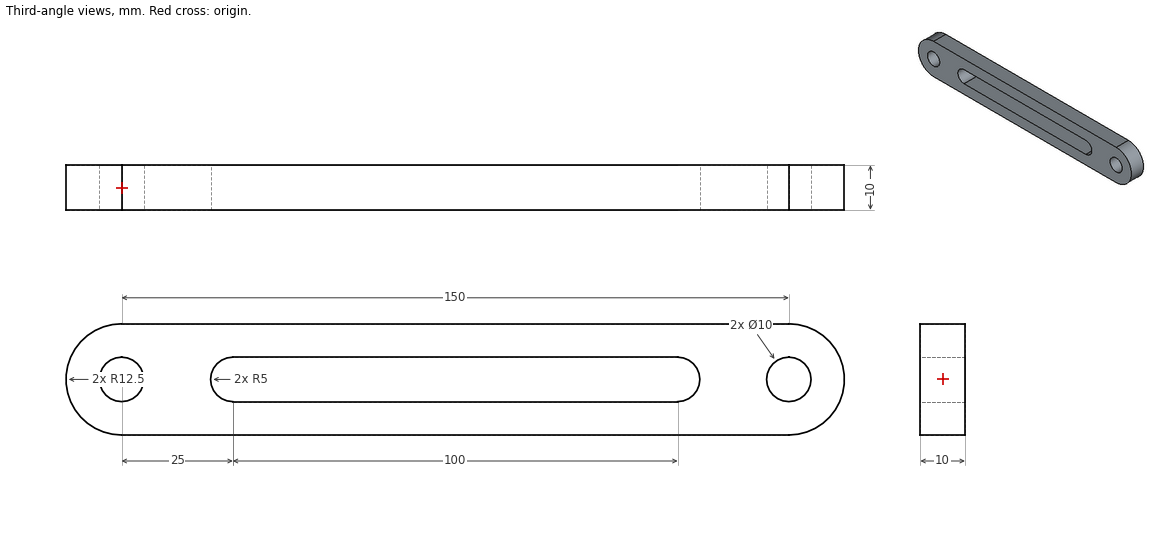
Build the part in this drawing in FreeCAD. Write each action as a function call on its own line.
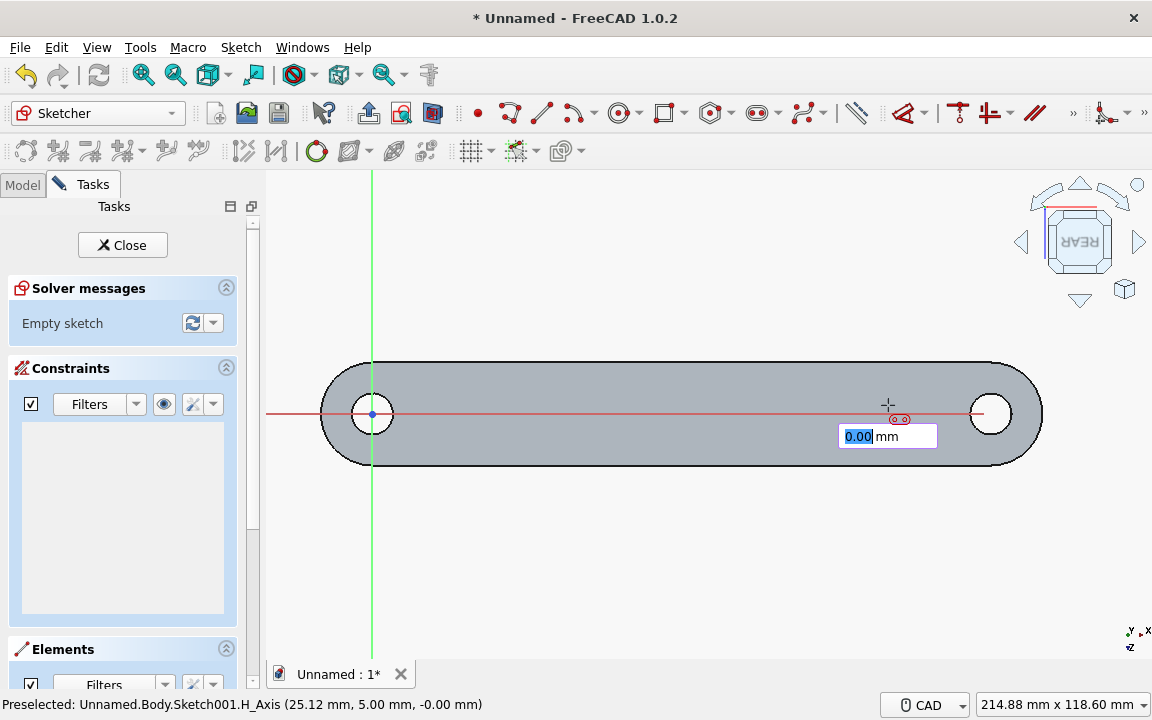
click(682, 393)
key(Escape)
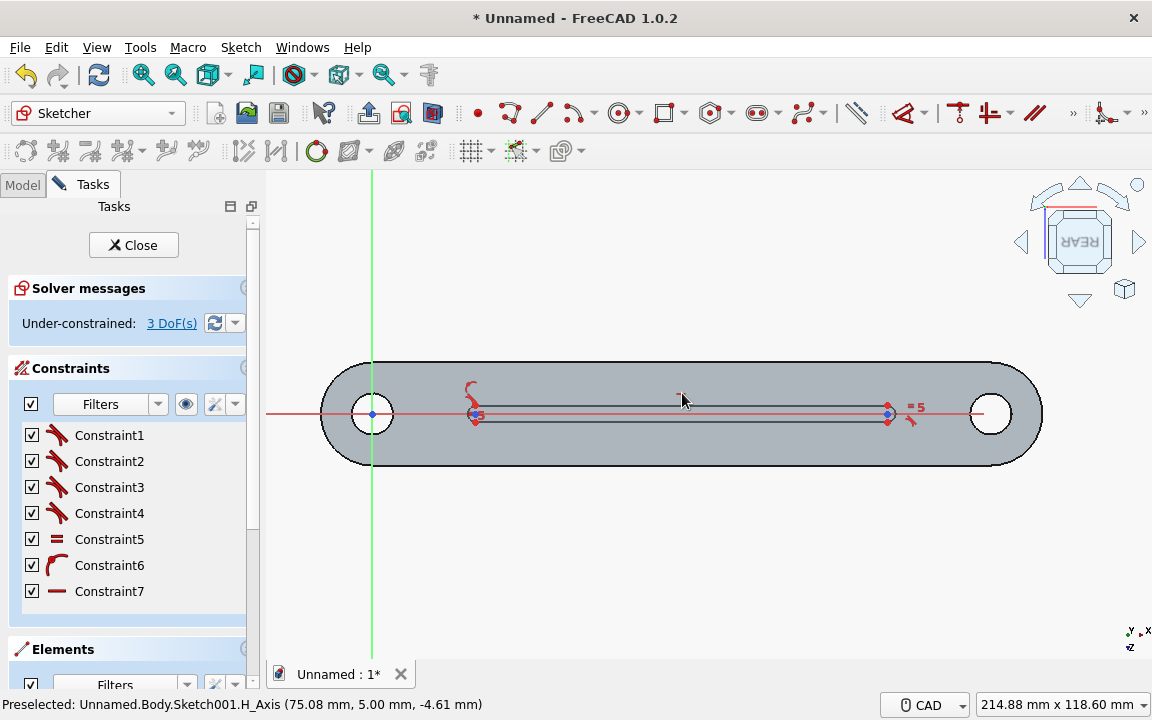
key(d)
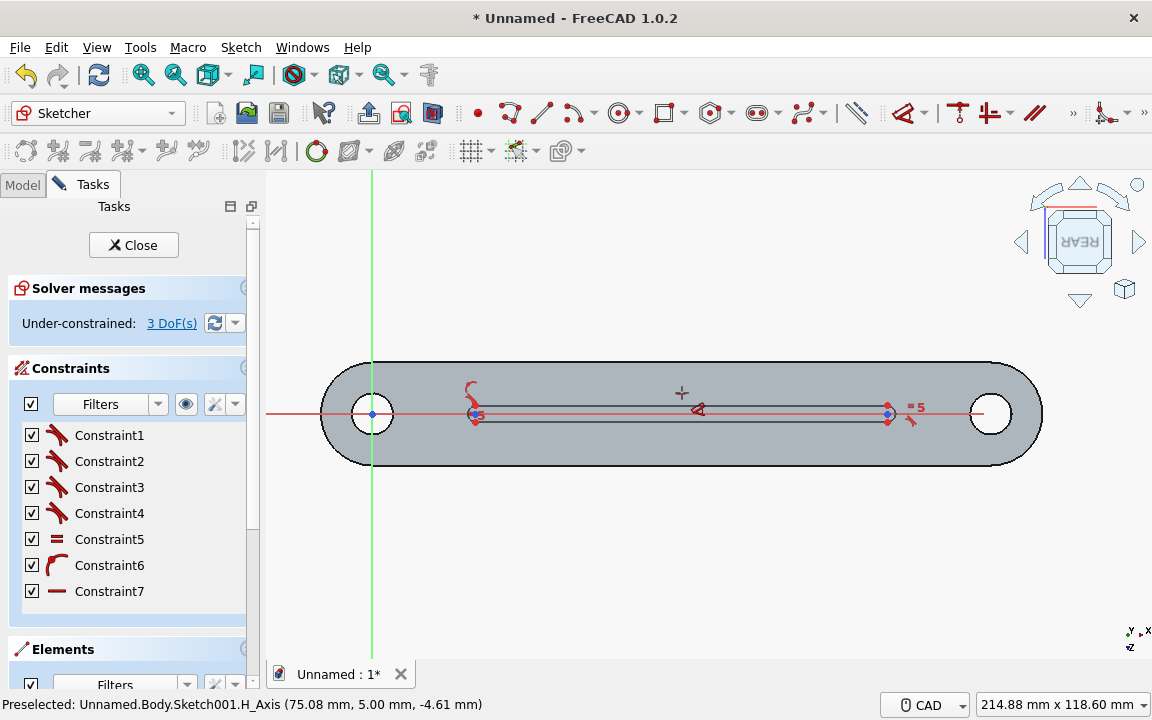
scroll(468, 414, up, 4)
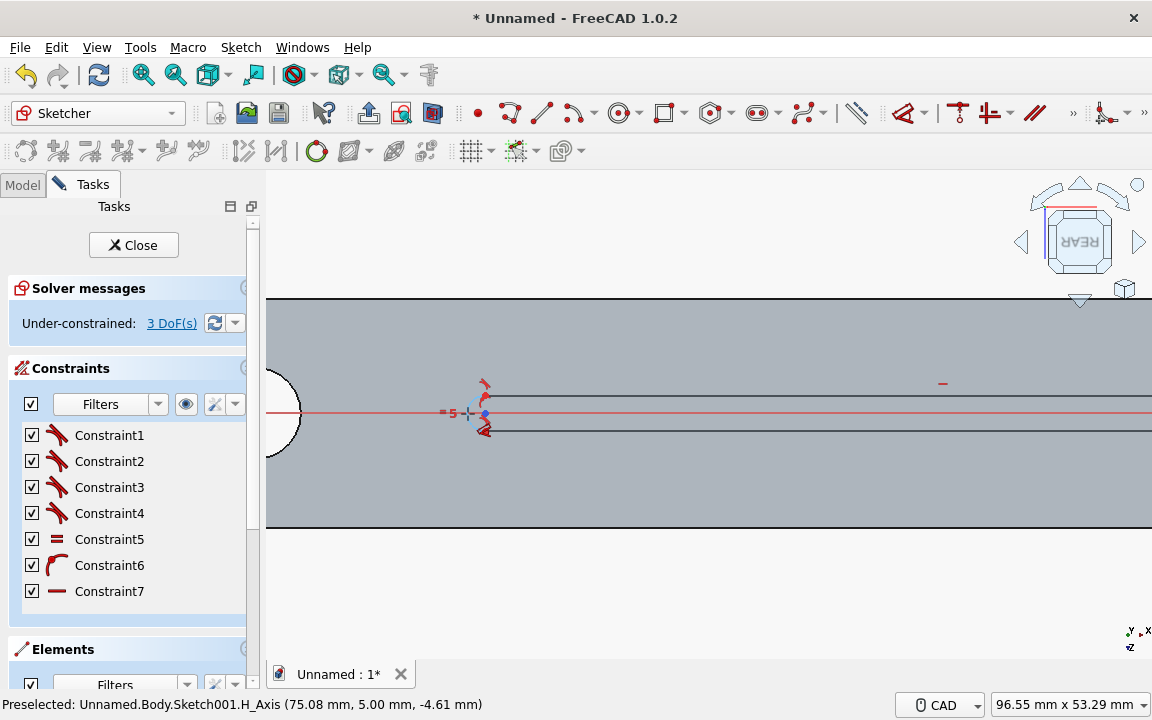
click(467, 413)
click(442, 388)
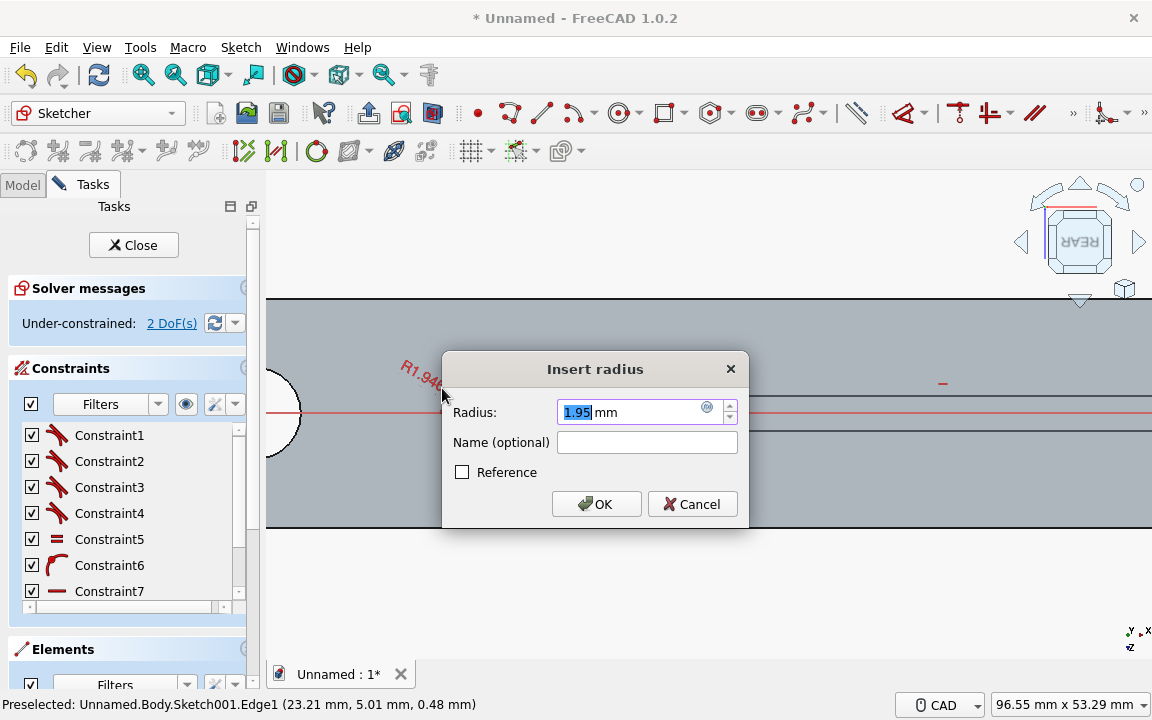
text(5)
key(Return)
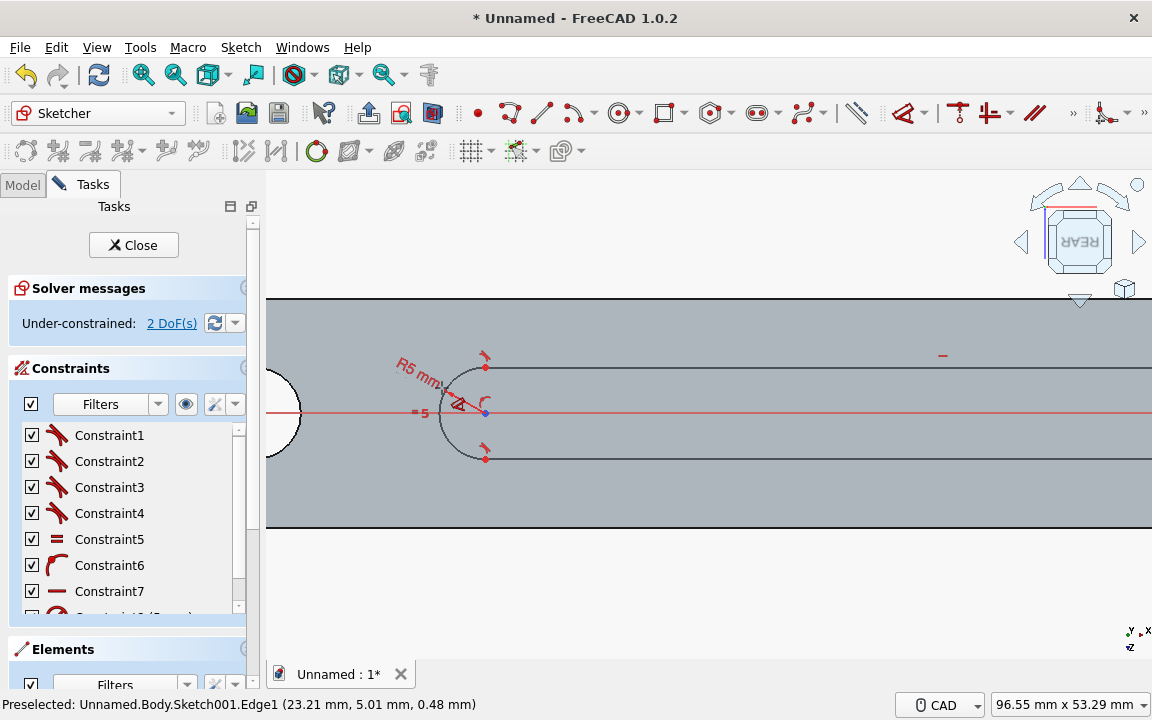
click(760, 368)
click(736, 334)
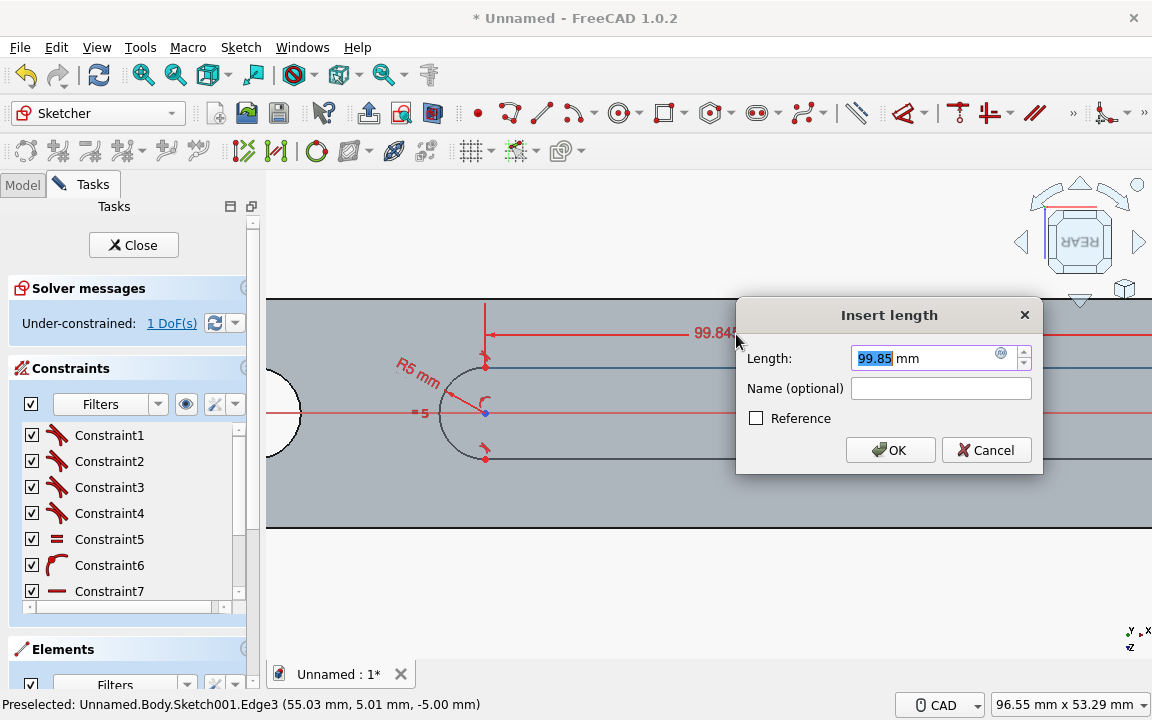
text(100)
key(Return)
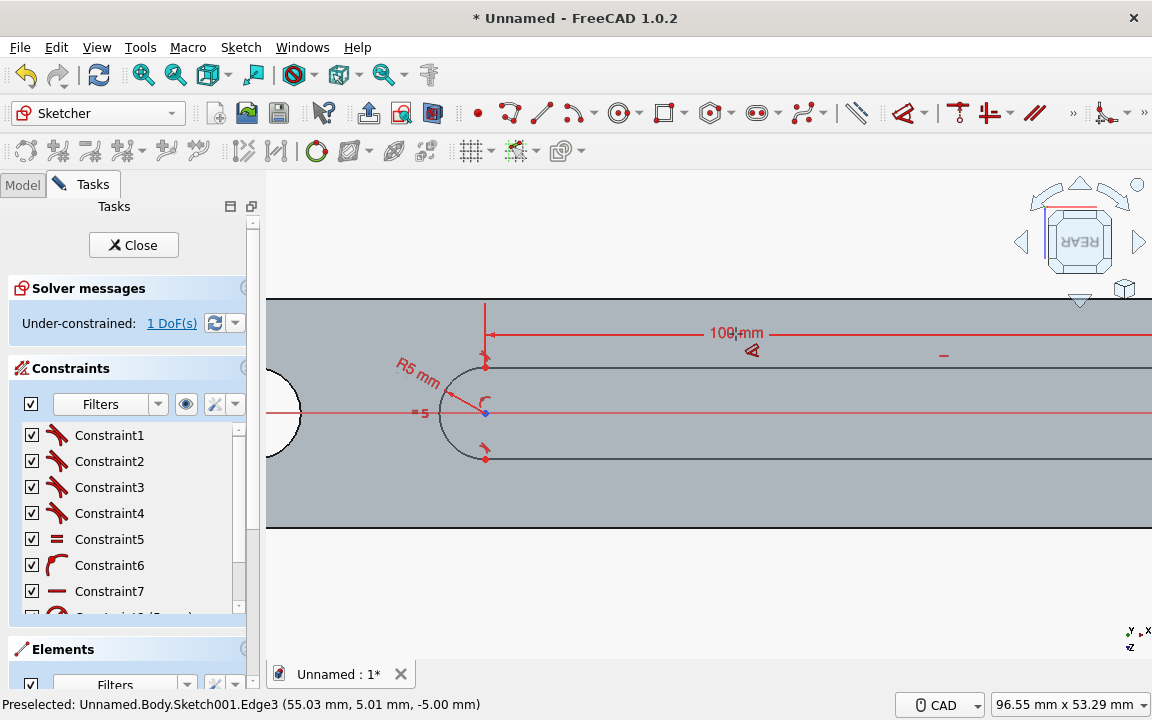
click(485, 368)
click(390, 334)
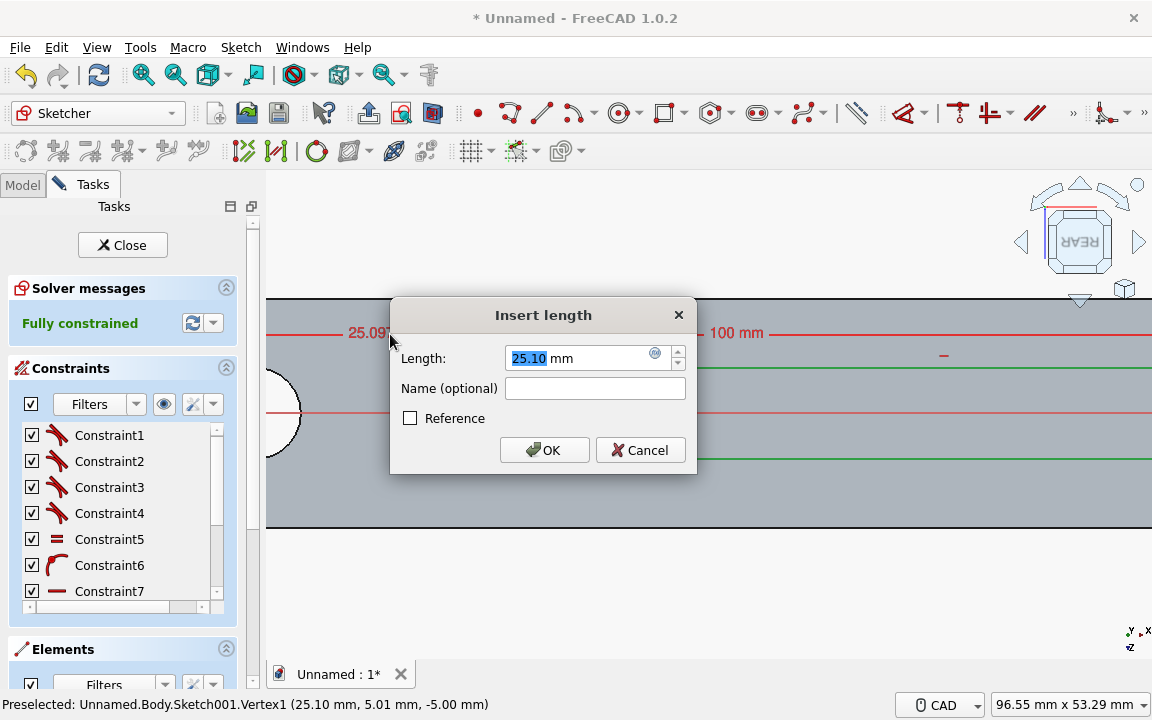
text(25)
key(Return)
key(Escape)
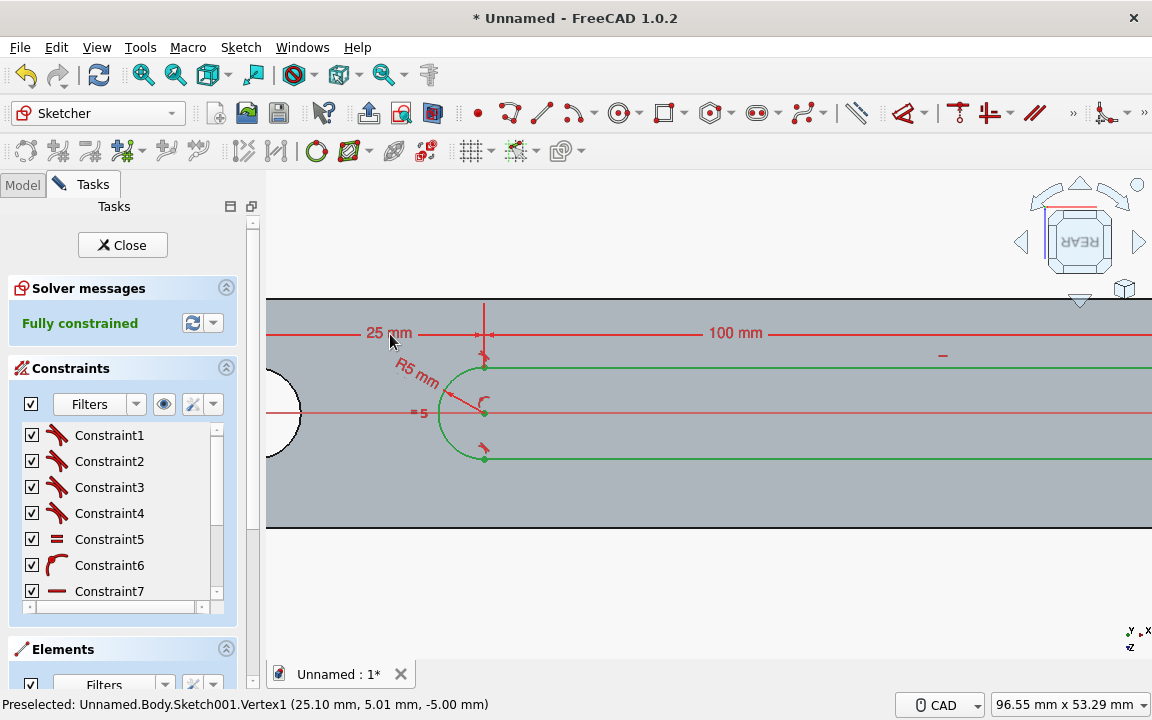
click(123, 245)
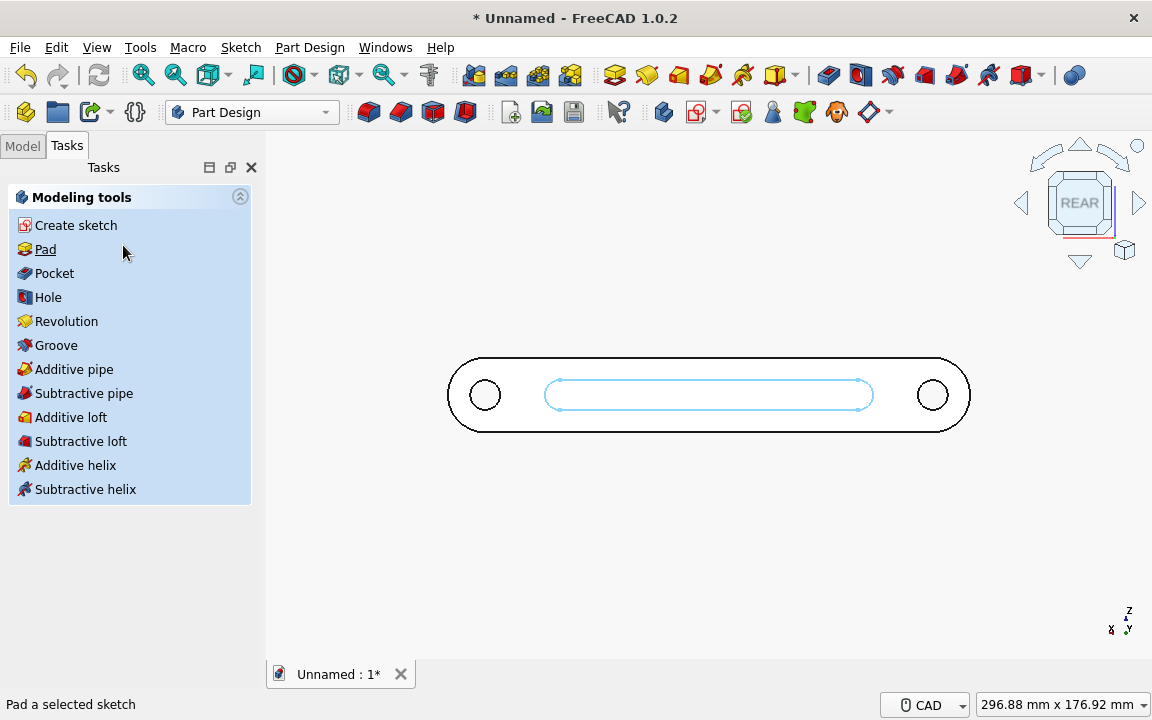
click(830, 76)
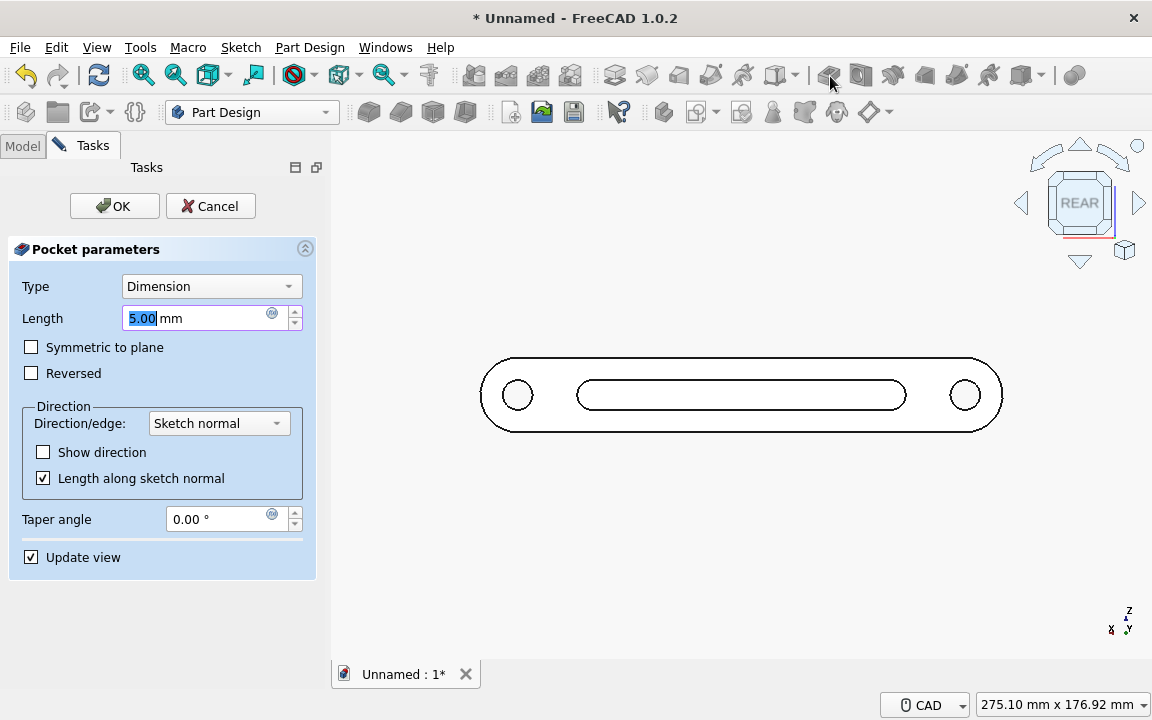
text(10)
key(Tab)